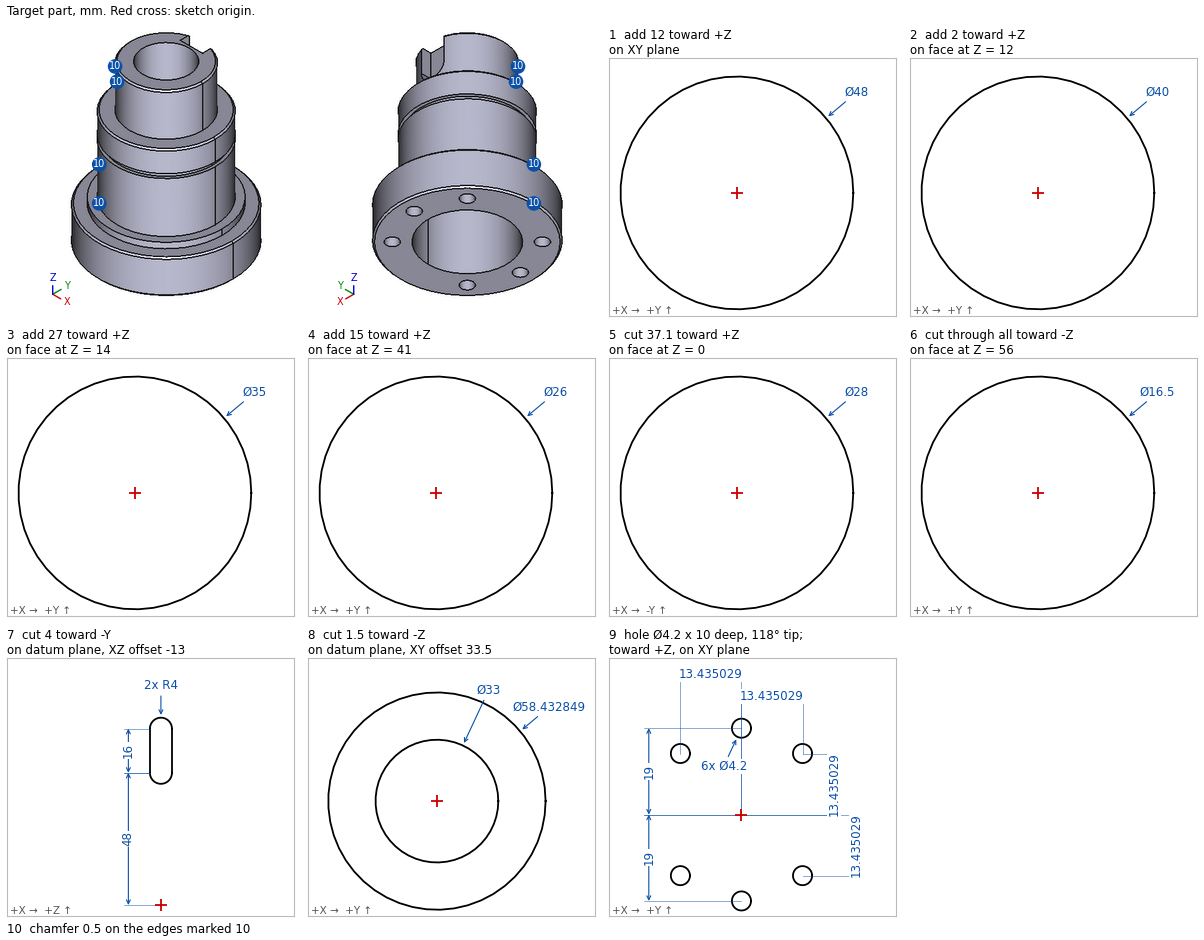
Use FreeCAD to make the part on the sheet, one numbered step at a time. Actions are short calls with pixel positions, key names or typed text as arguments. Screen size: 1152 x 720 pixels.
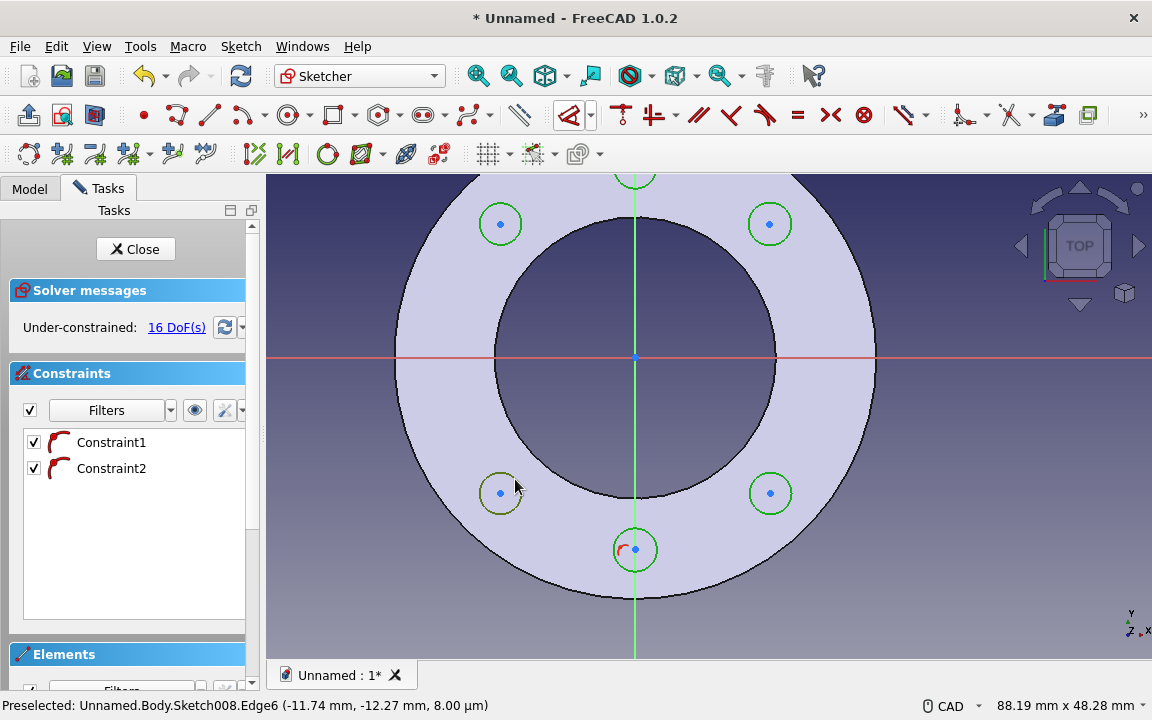
click(798, 116)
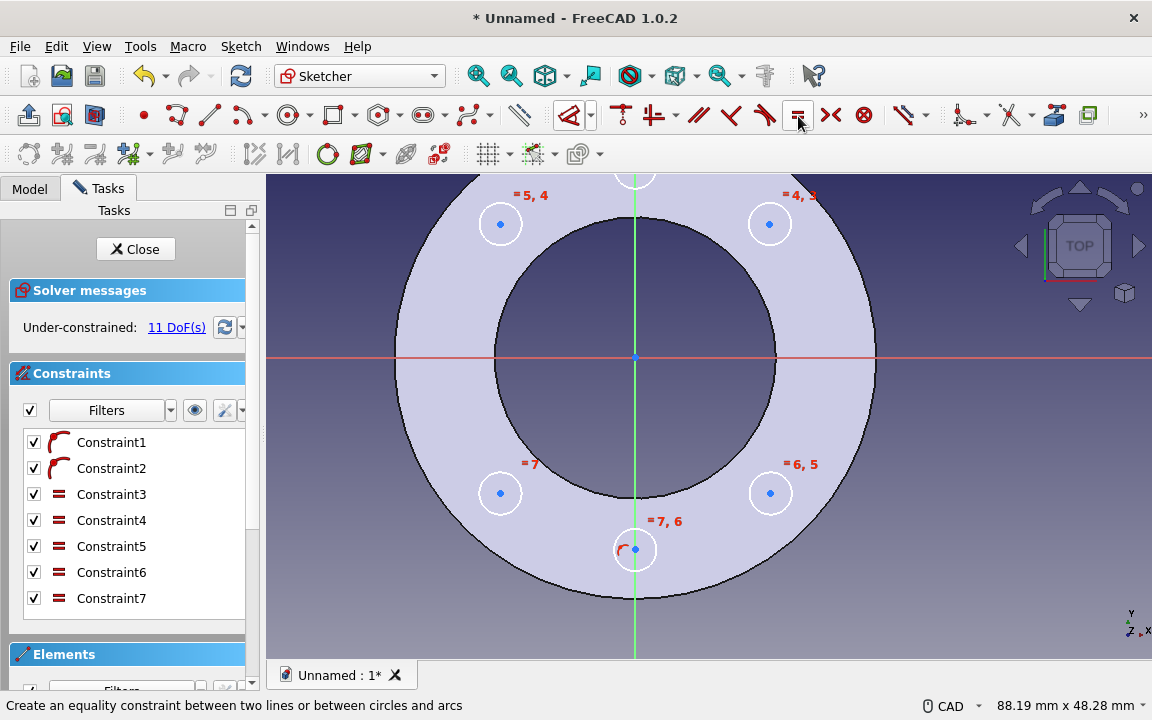
click(770, 224)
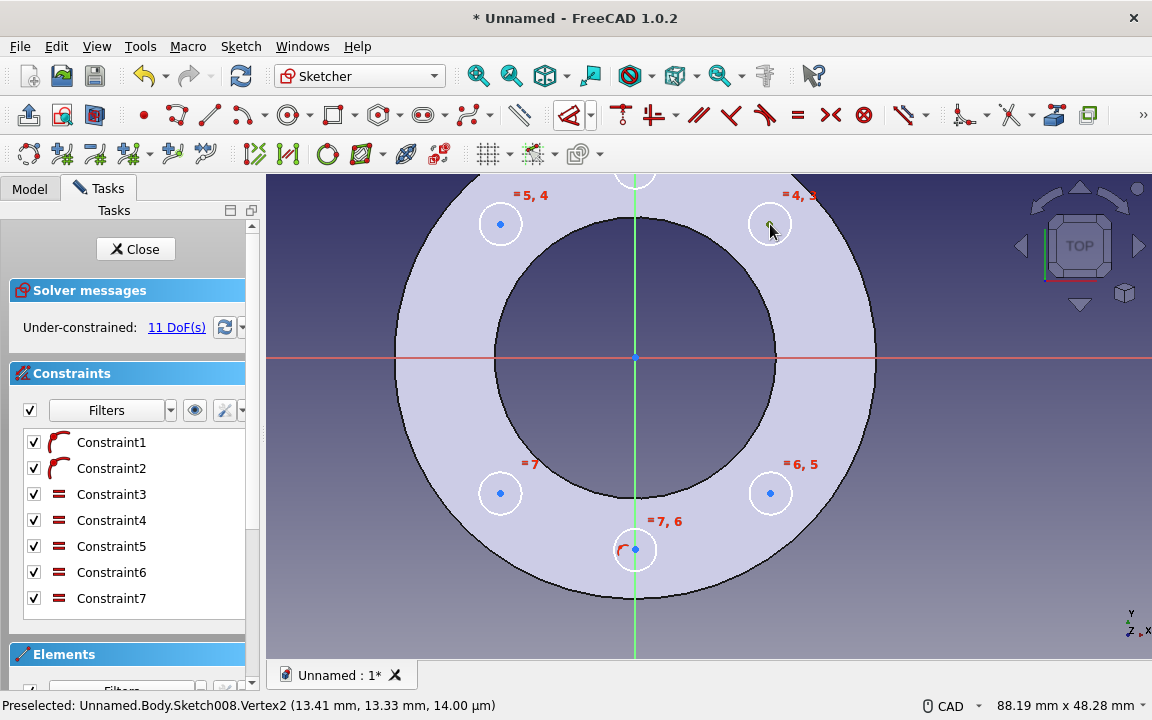
click(501, 224)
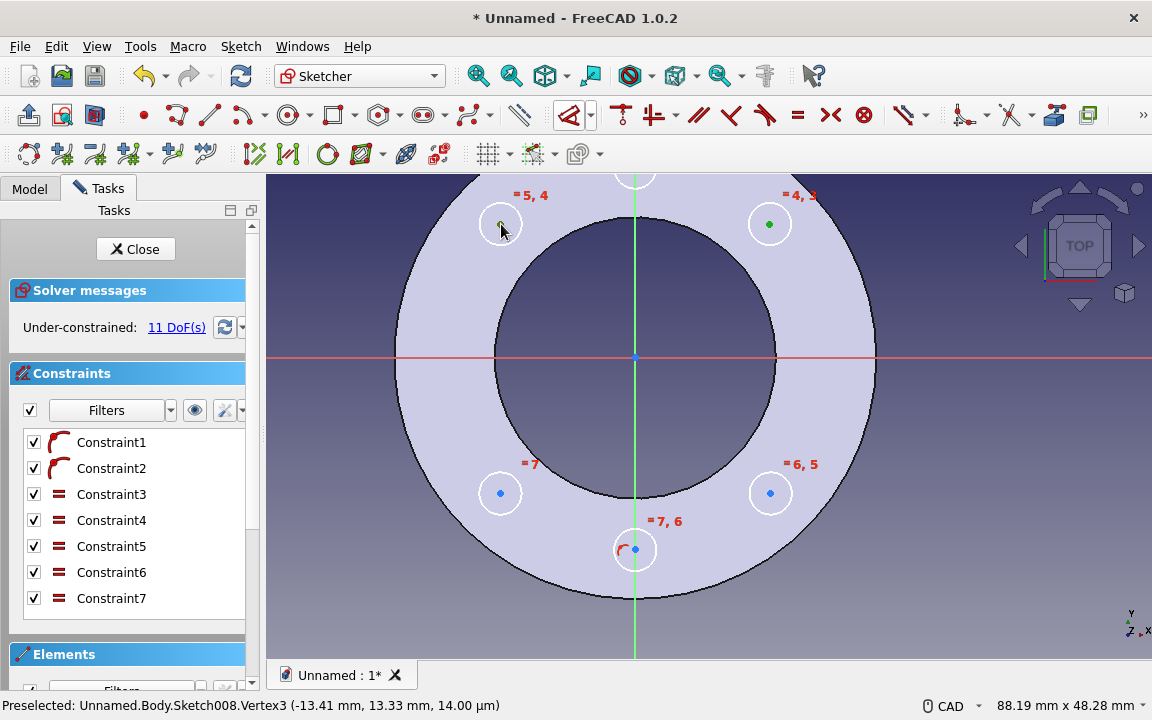
key(h)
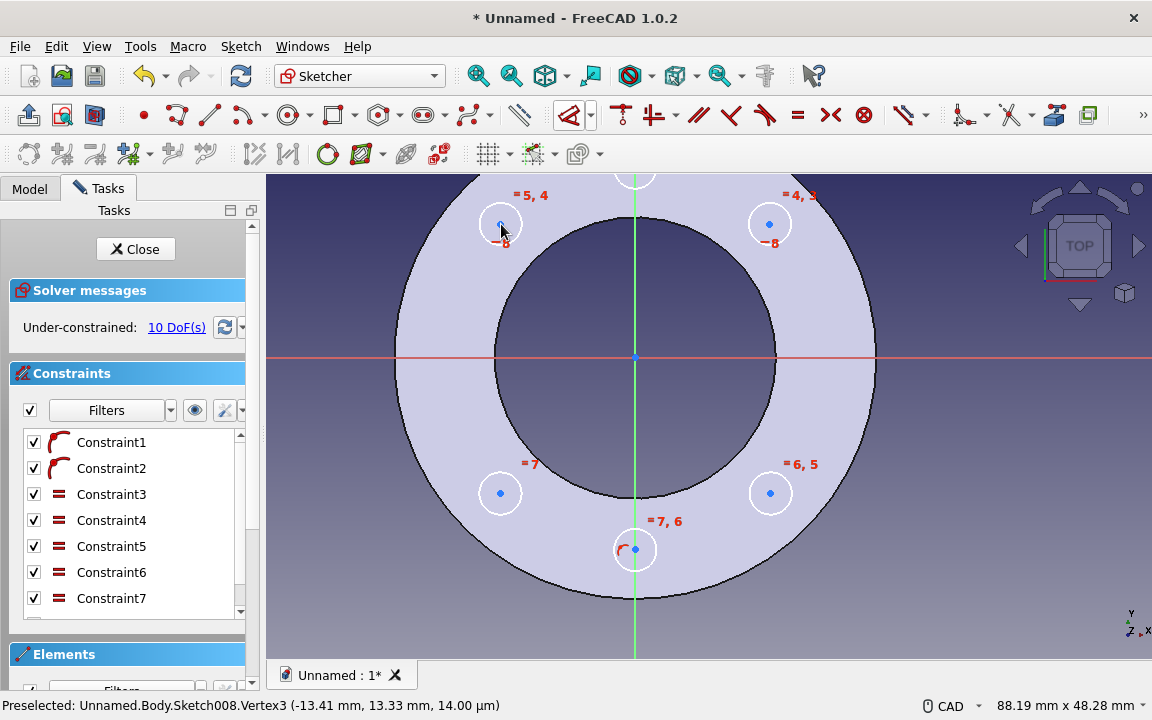
click(770, 224)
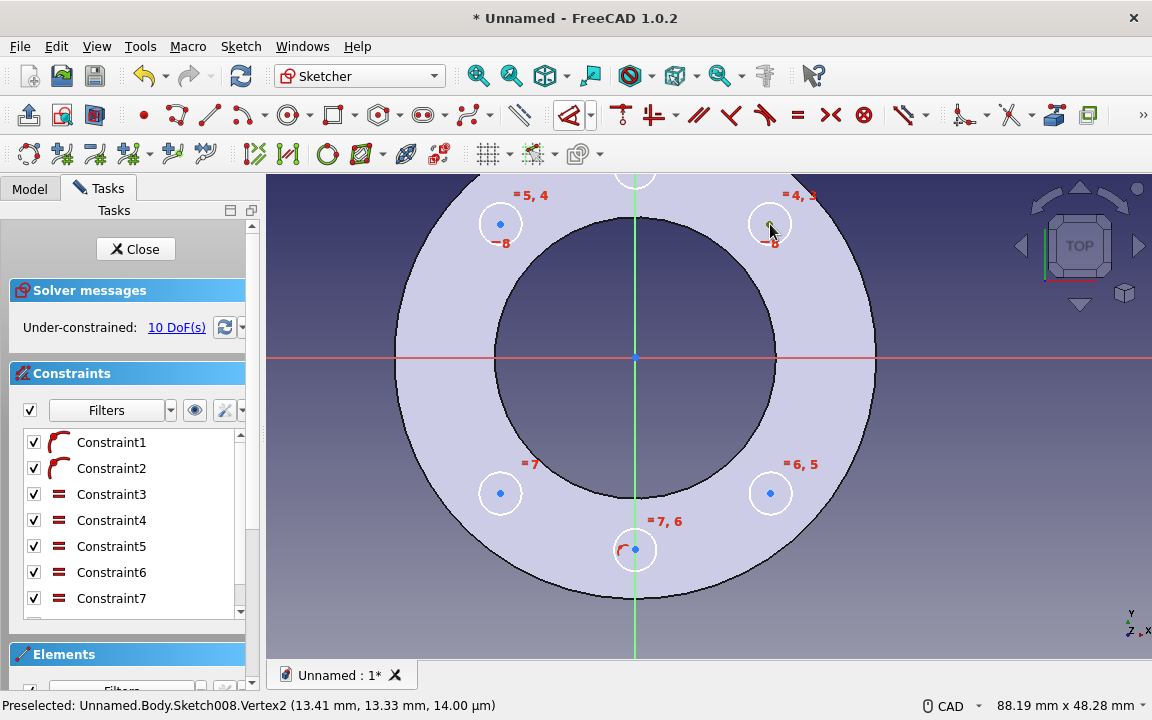
click(771, 494)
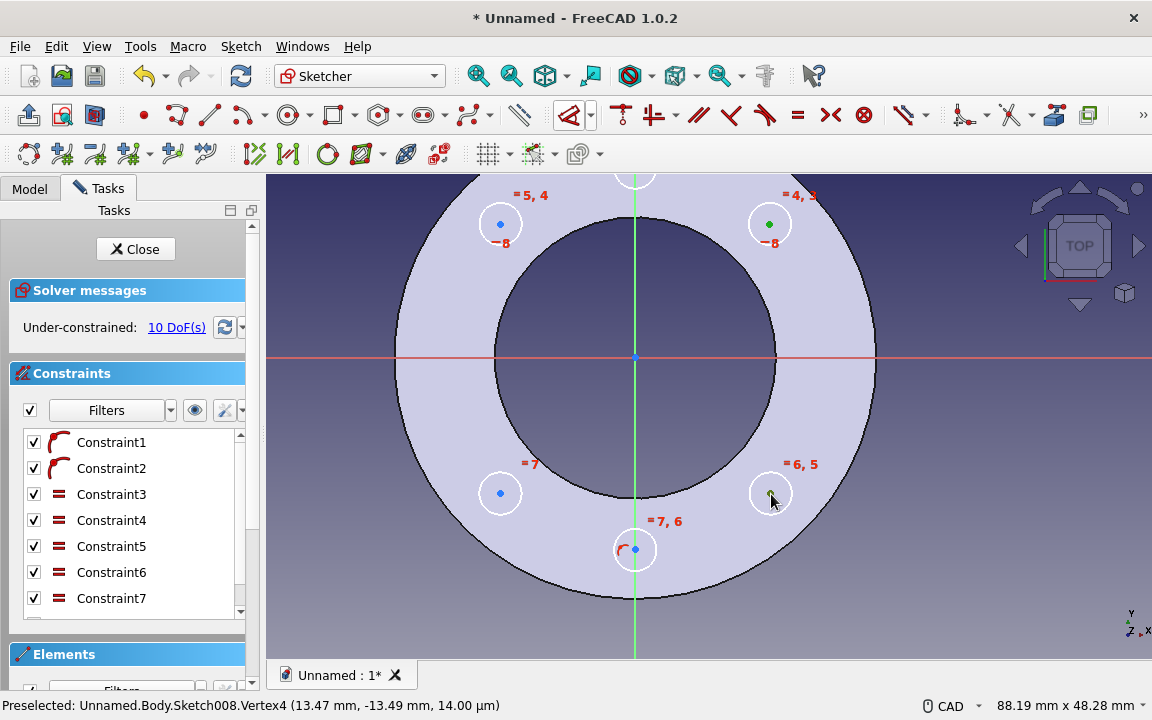
click(676, 116)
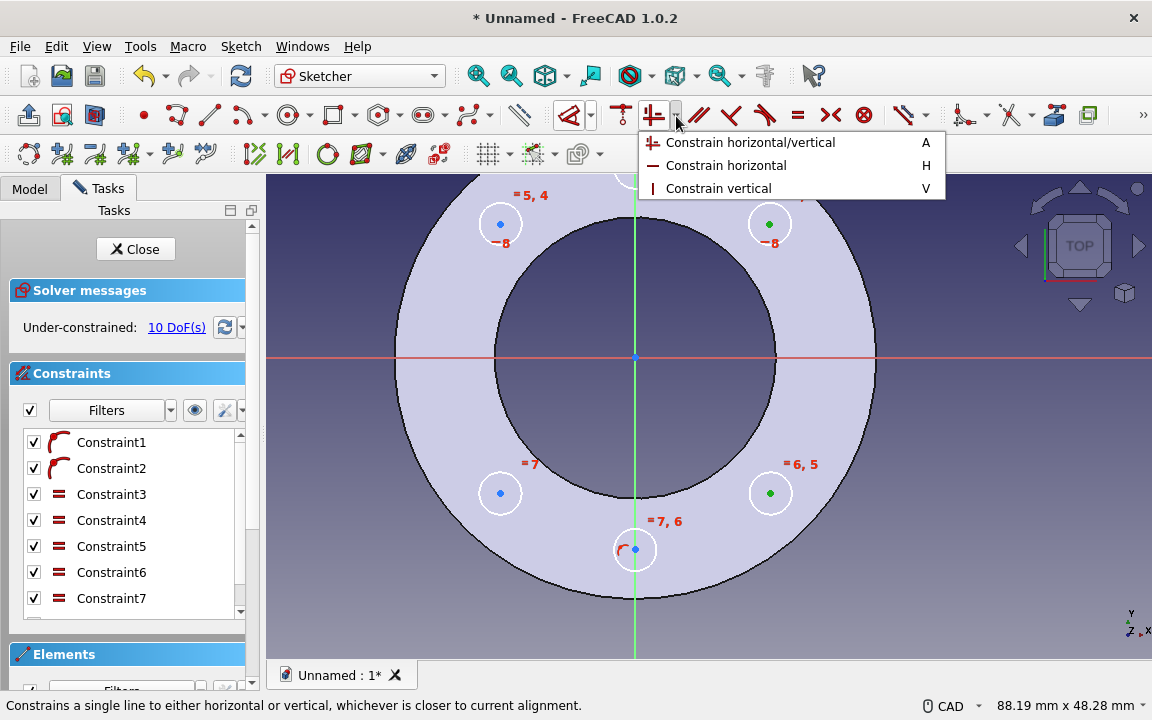
click(792, 188)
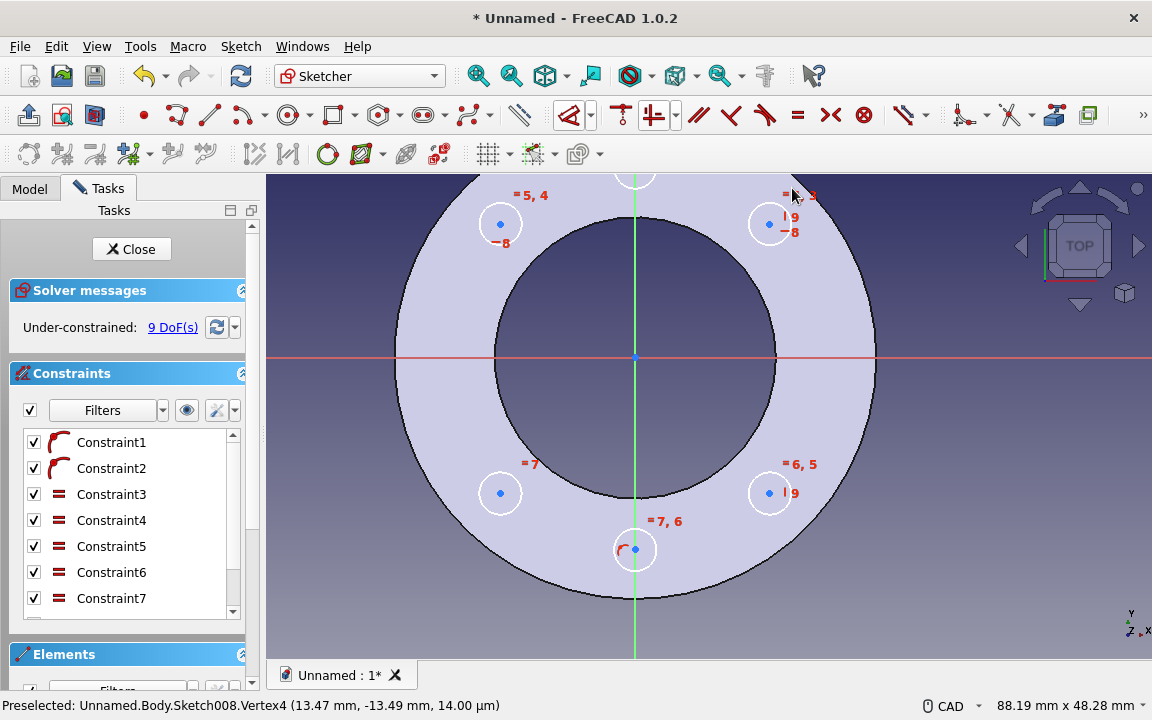
click(501, 224)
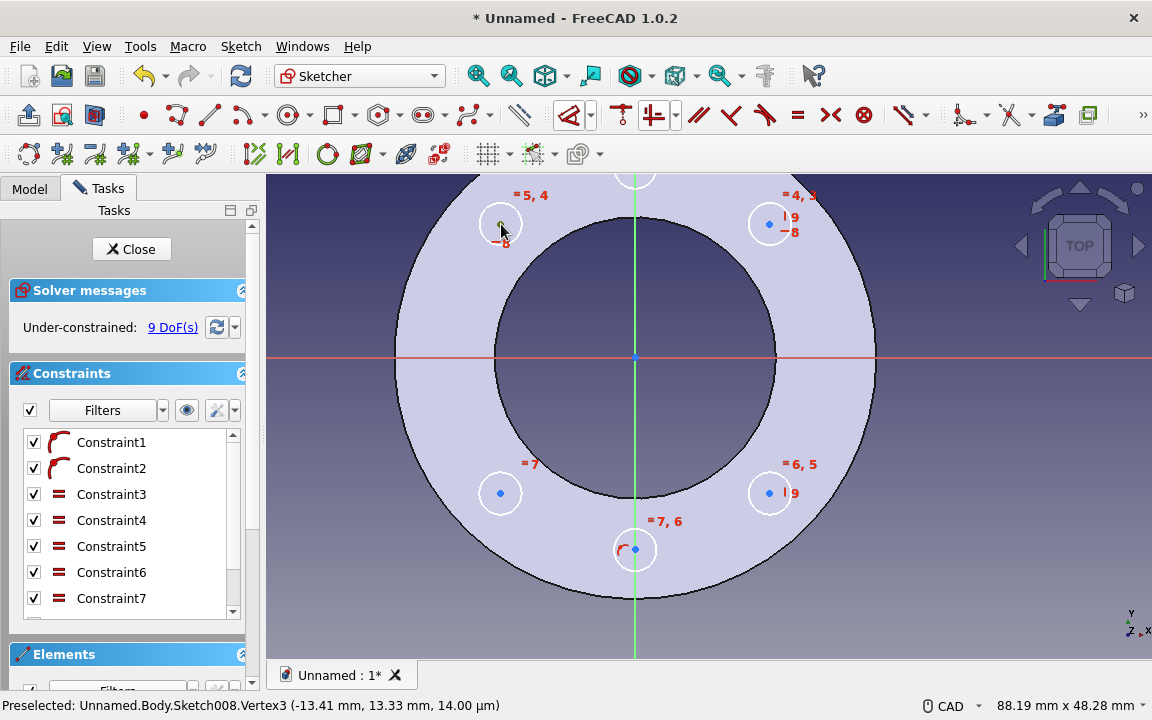
click(500, 494)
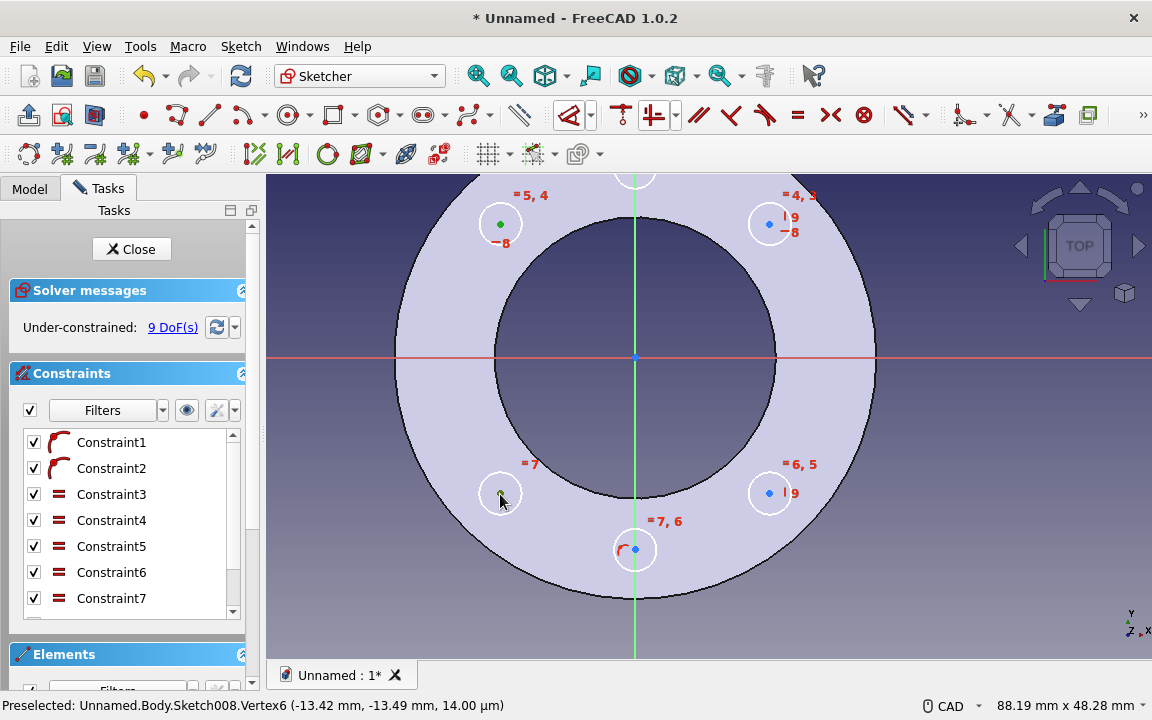
click(676, 116)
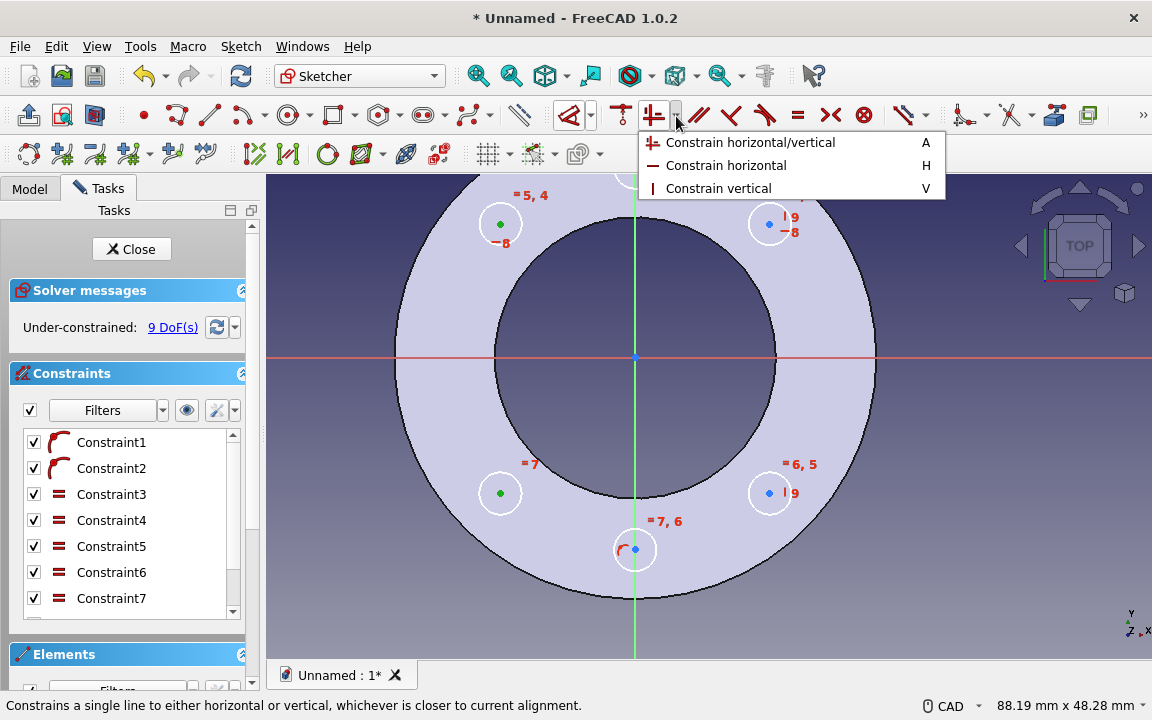
click(792, 188)